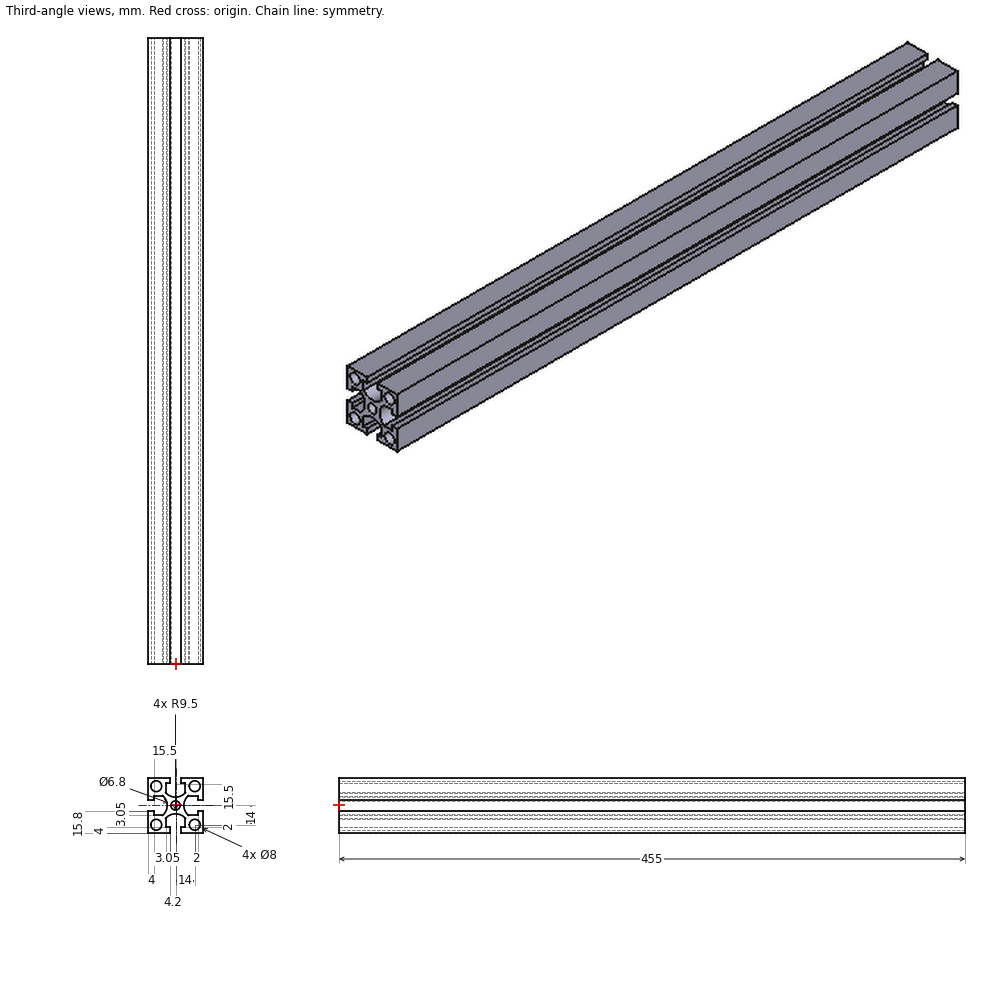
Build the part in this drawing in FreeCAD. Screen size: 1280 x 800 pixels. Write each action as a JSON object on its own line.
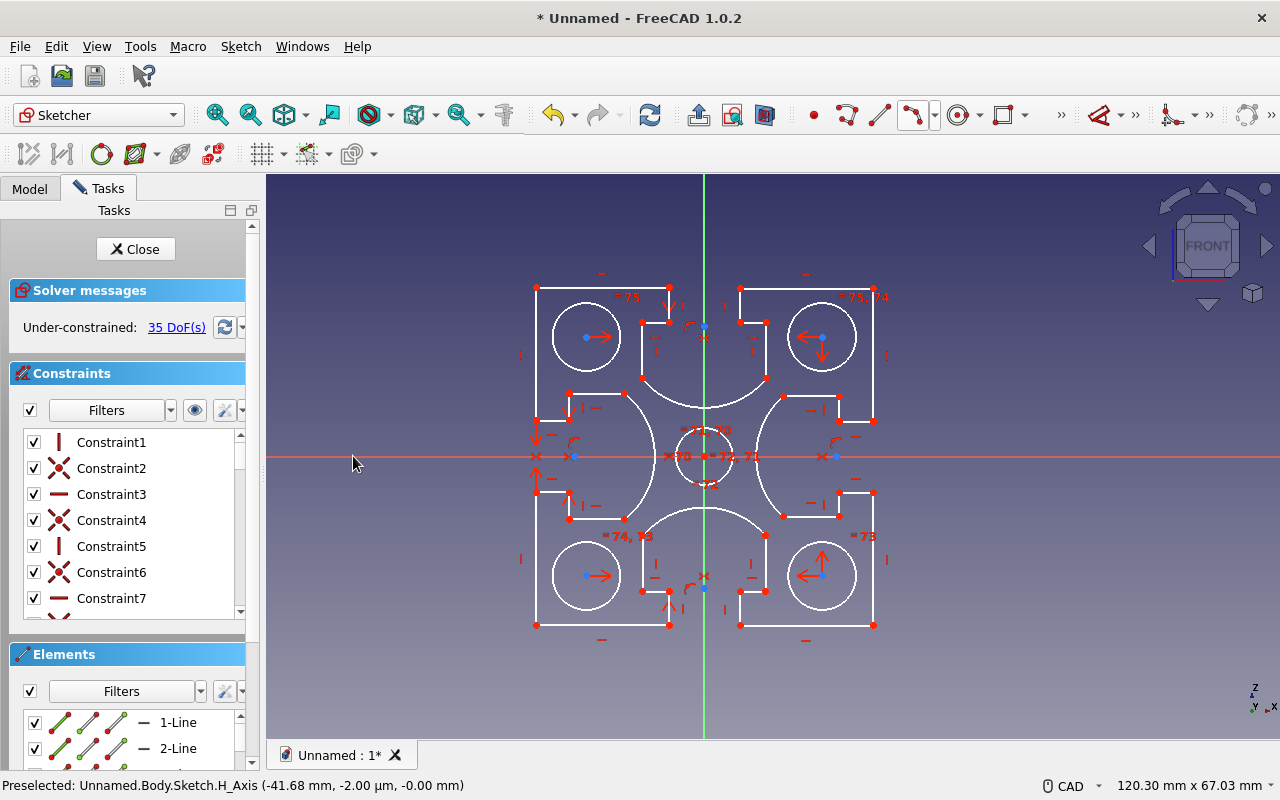
{"action": "left_click", "coordinate": [643, 592]}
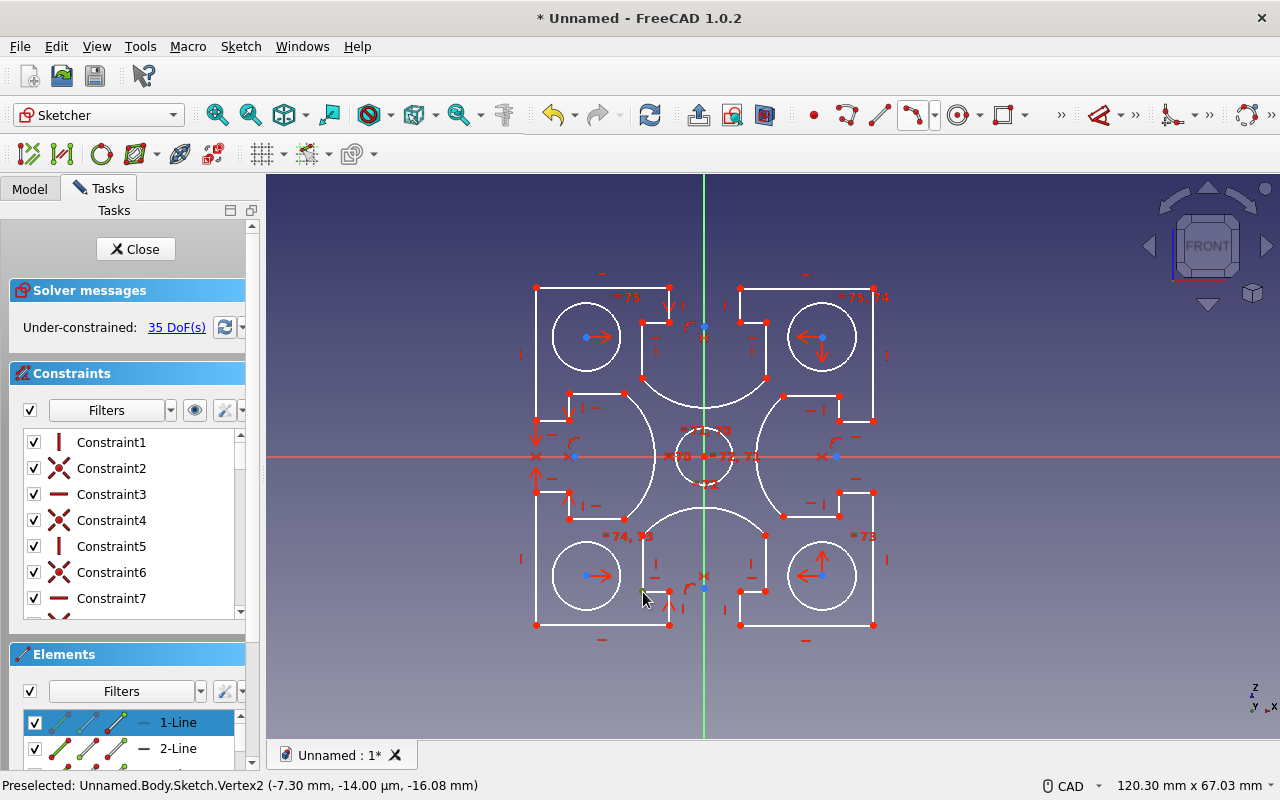
{"action": "left_click", "coordinate": [642, 323]}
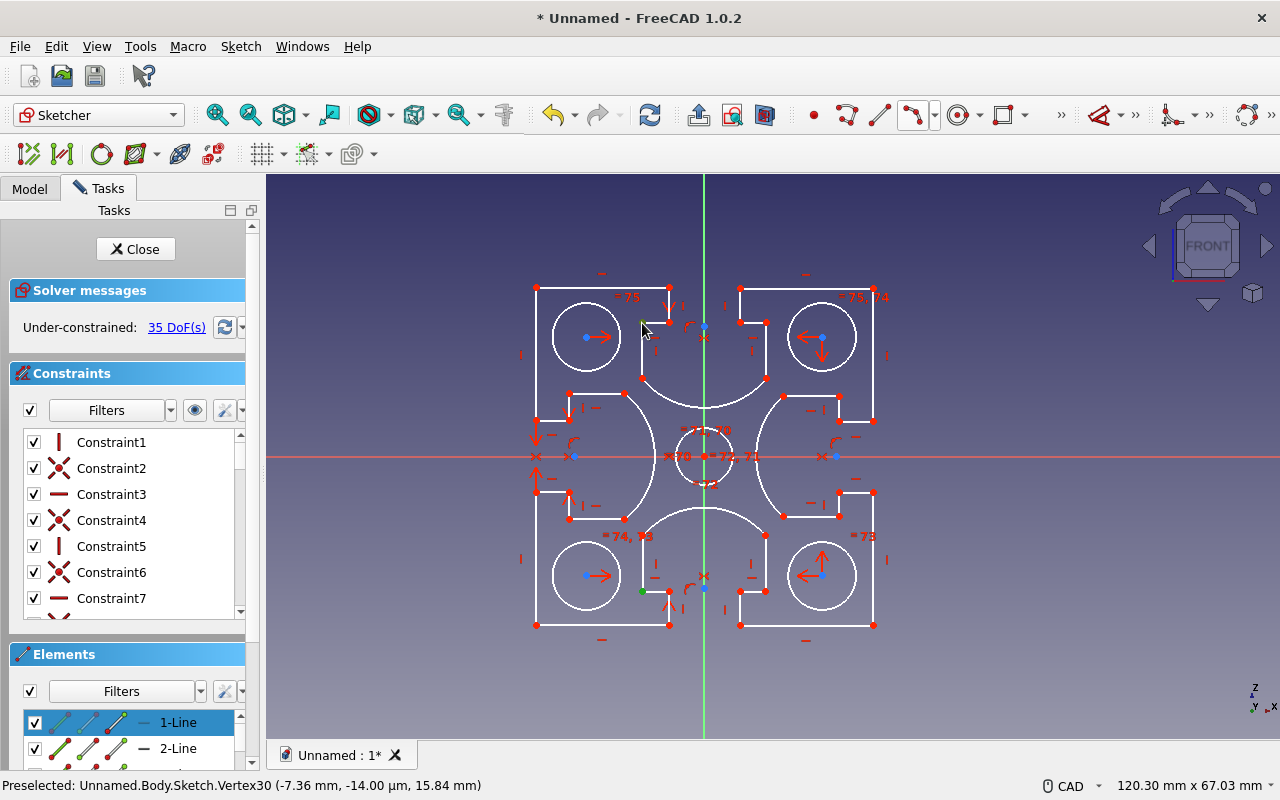
{"action": "left_click", "coordinate": [353, 456]}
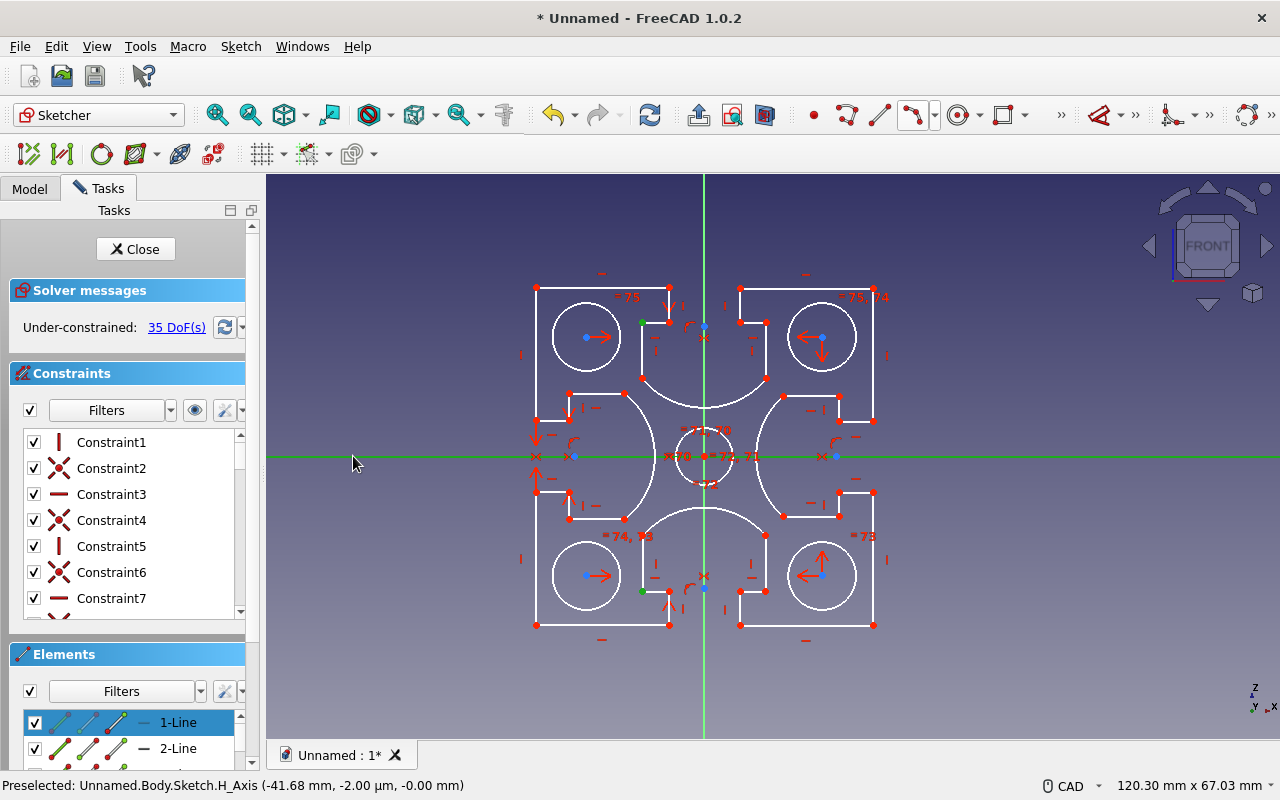
{"action": "key", "text": "s"}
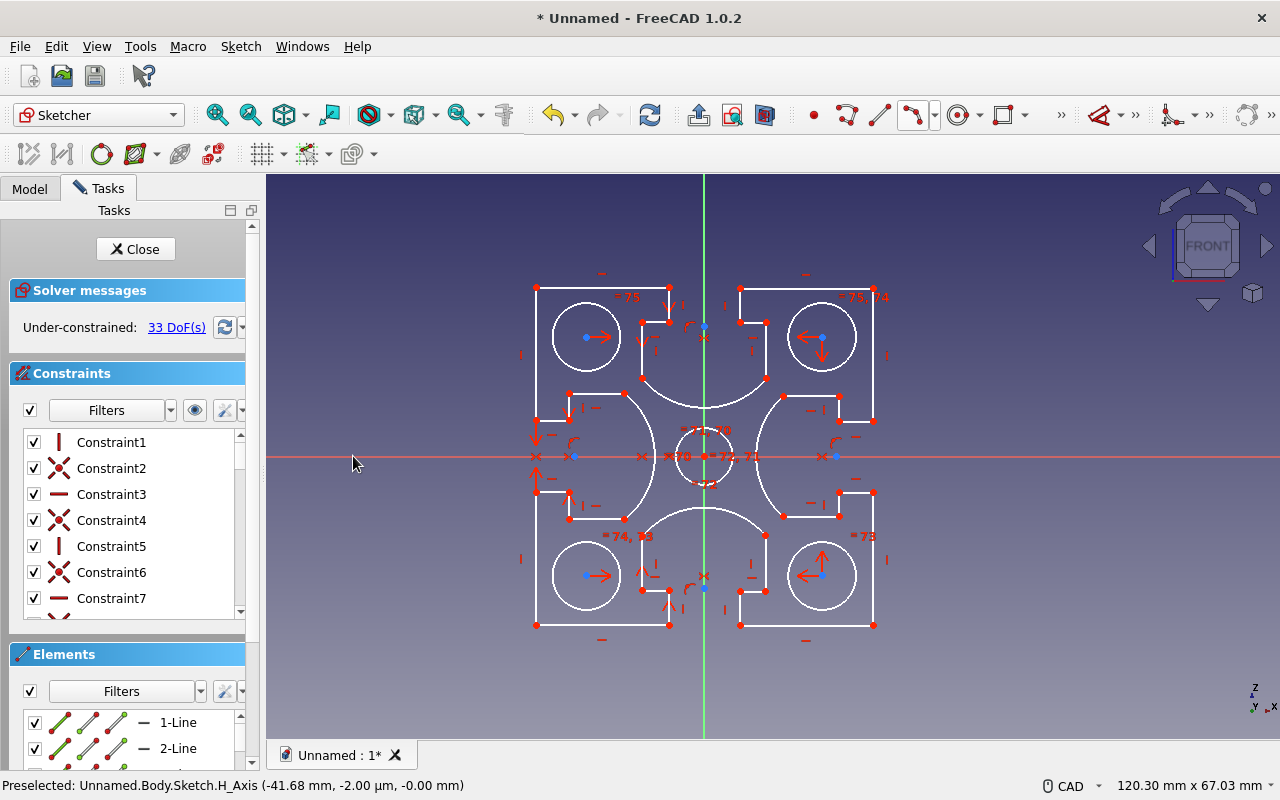
{"action": "left_click", "coordinate": [642, 322]}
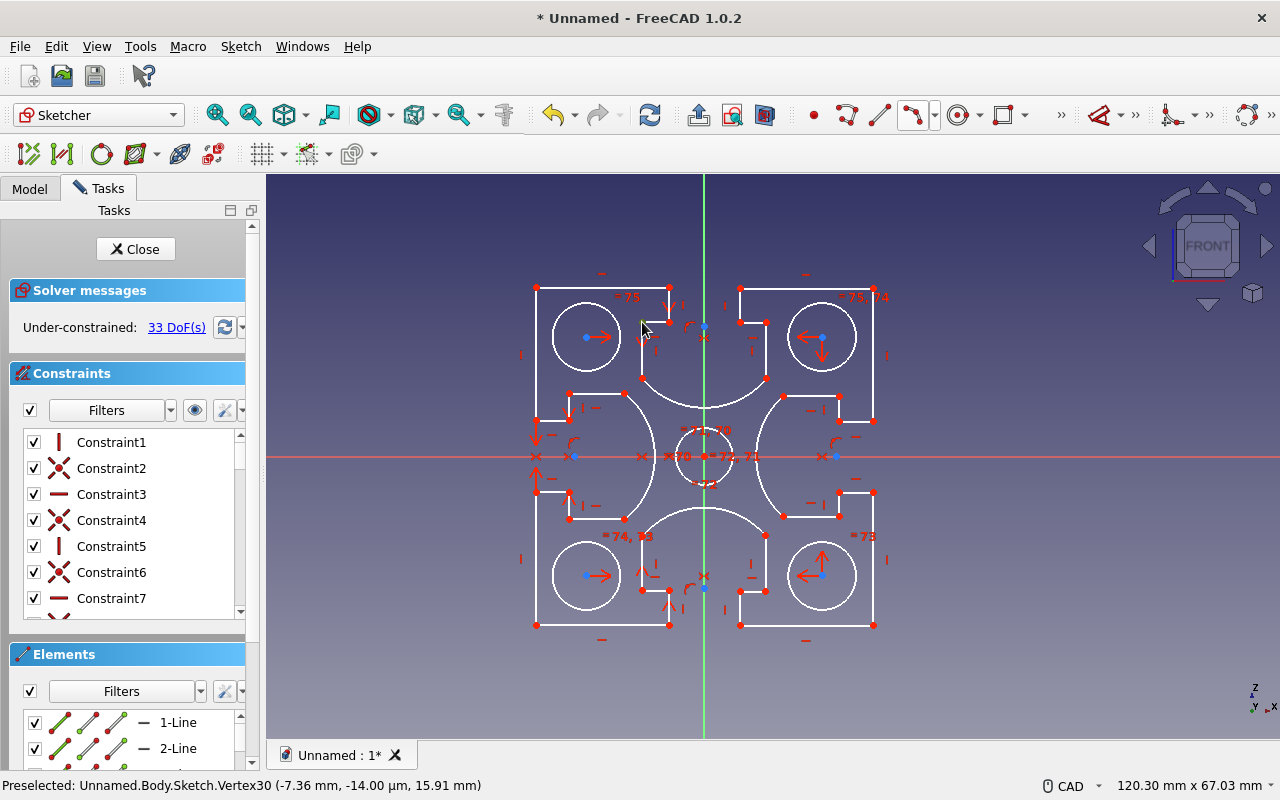
{"action": "left_click", "coordinate": [766, 323]}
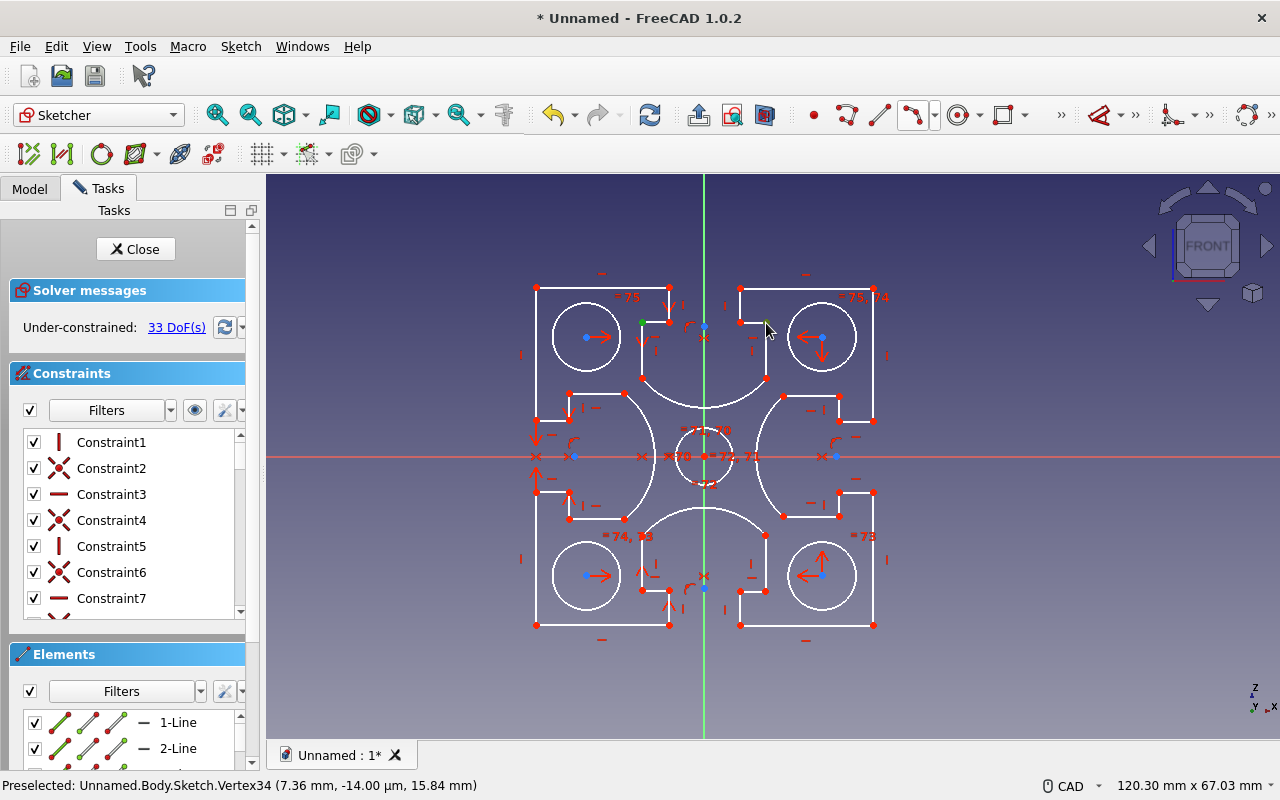
{"action": "left_click", "coordinate": [704, 675]}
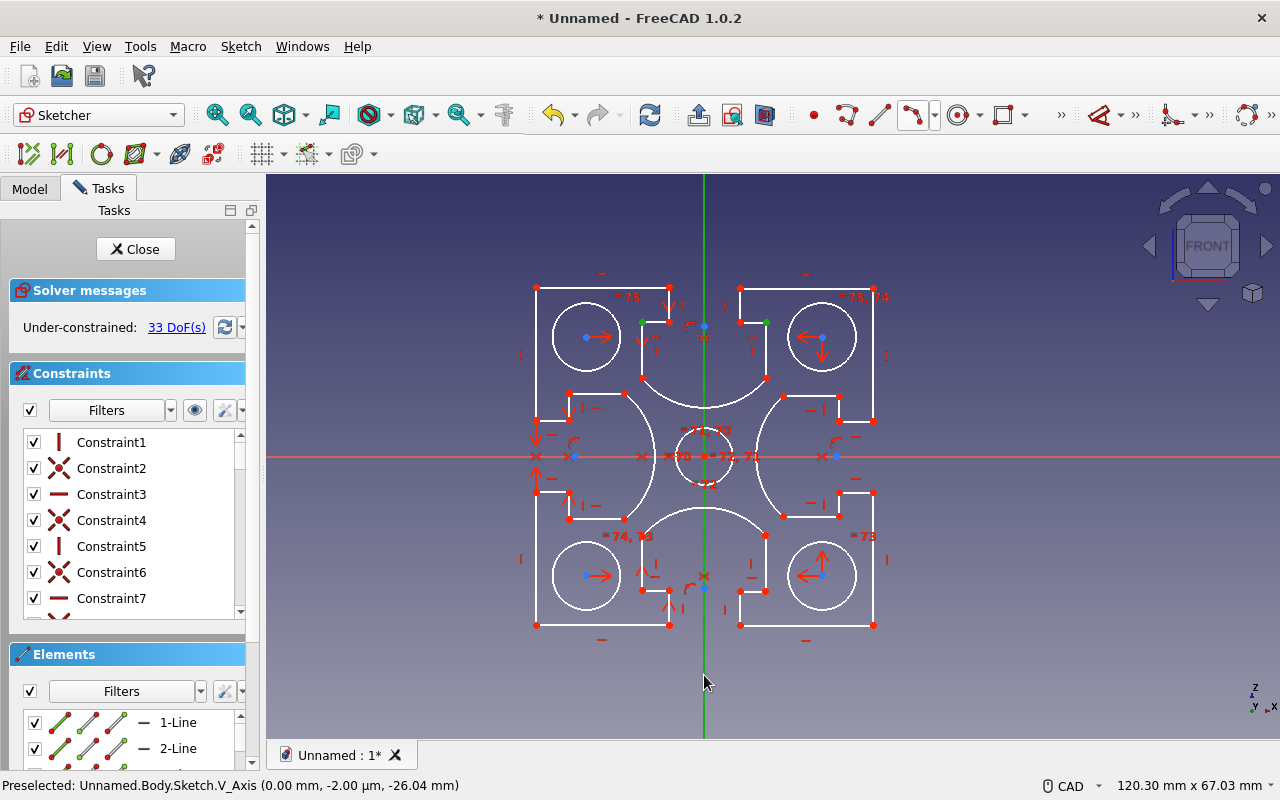
{"action": "key", "text": "s"}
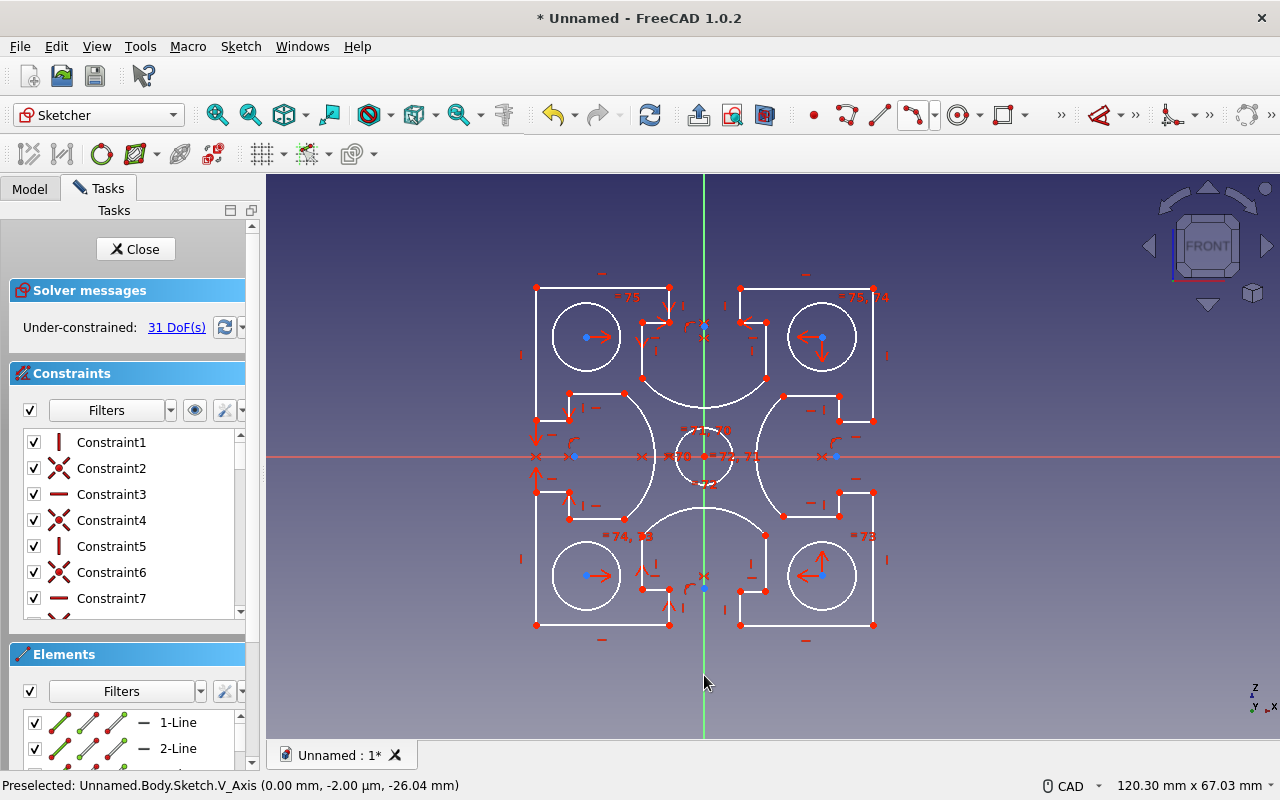
{"action": "left_click", "coordinate": [669, 288]}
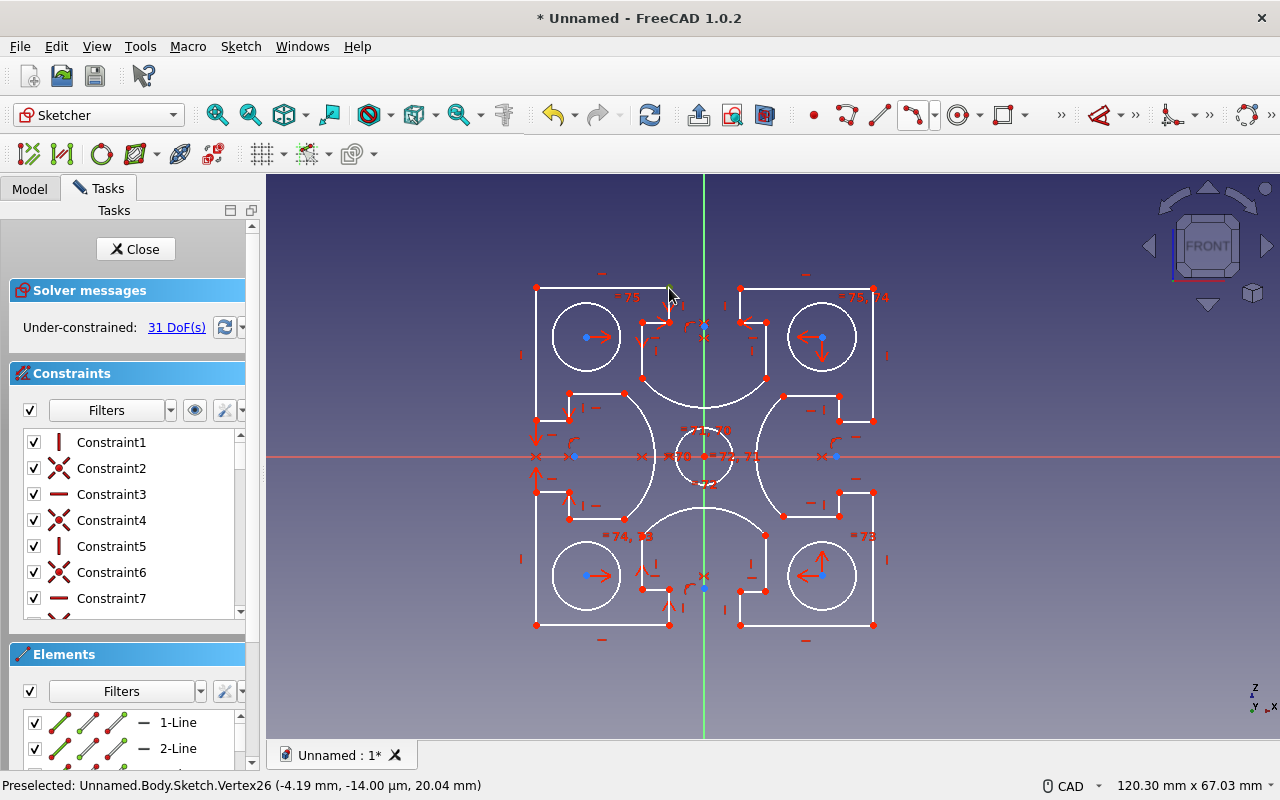
{"action": "left_click", "coordinate": [740, 289]}